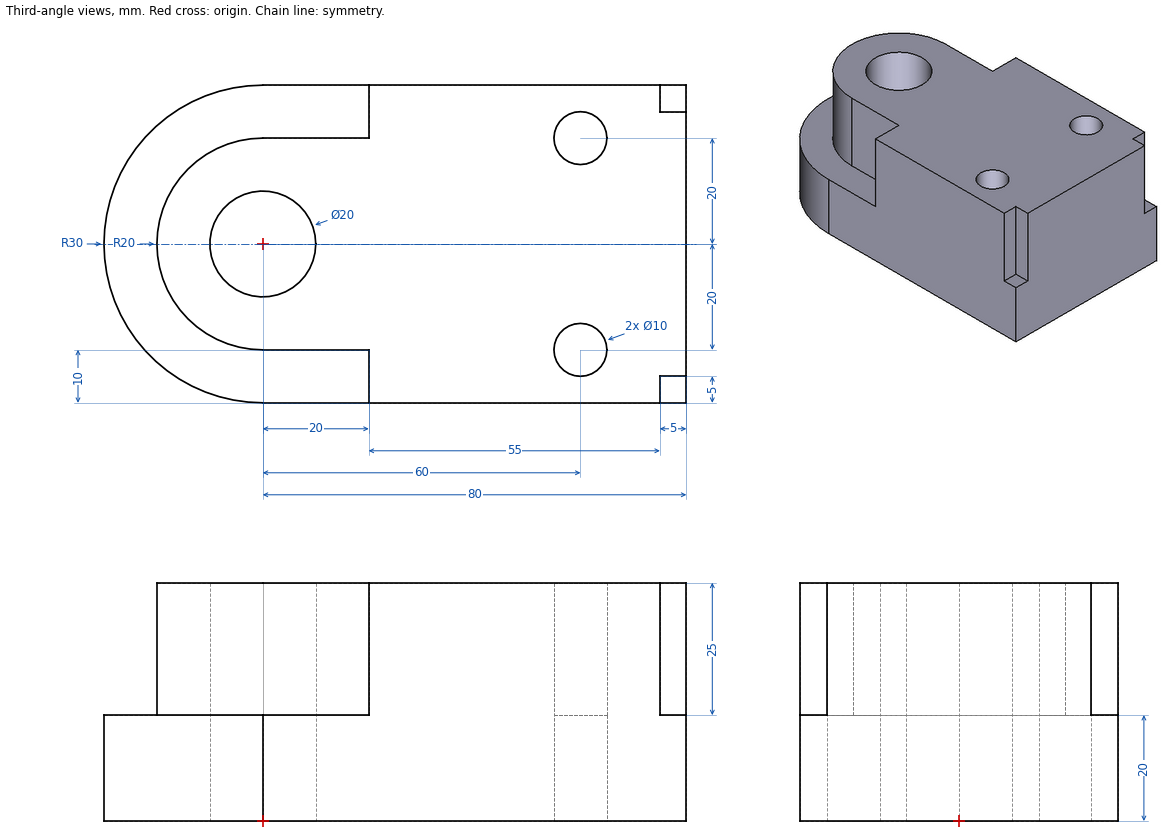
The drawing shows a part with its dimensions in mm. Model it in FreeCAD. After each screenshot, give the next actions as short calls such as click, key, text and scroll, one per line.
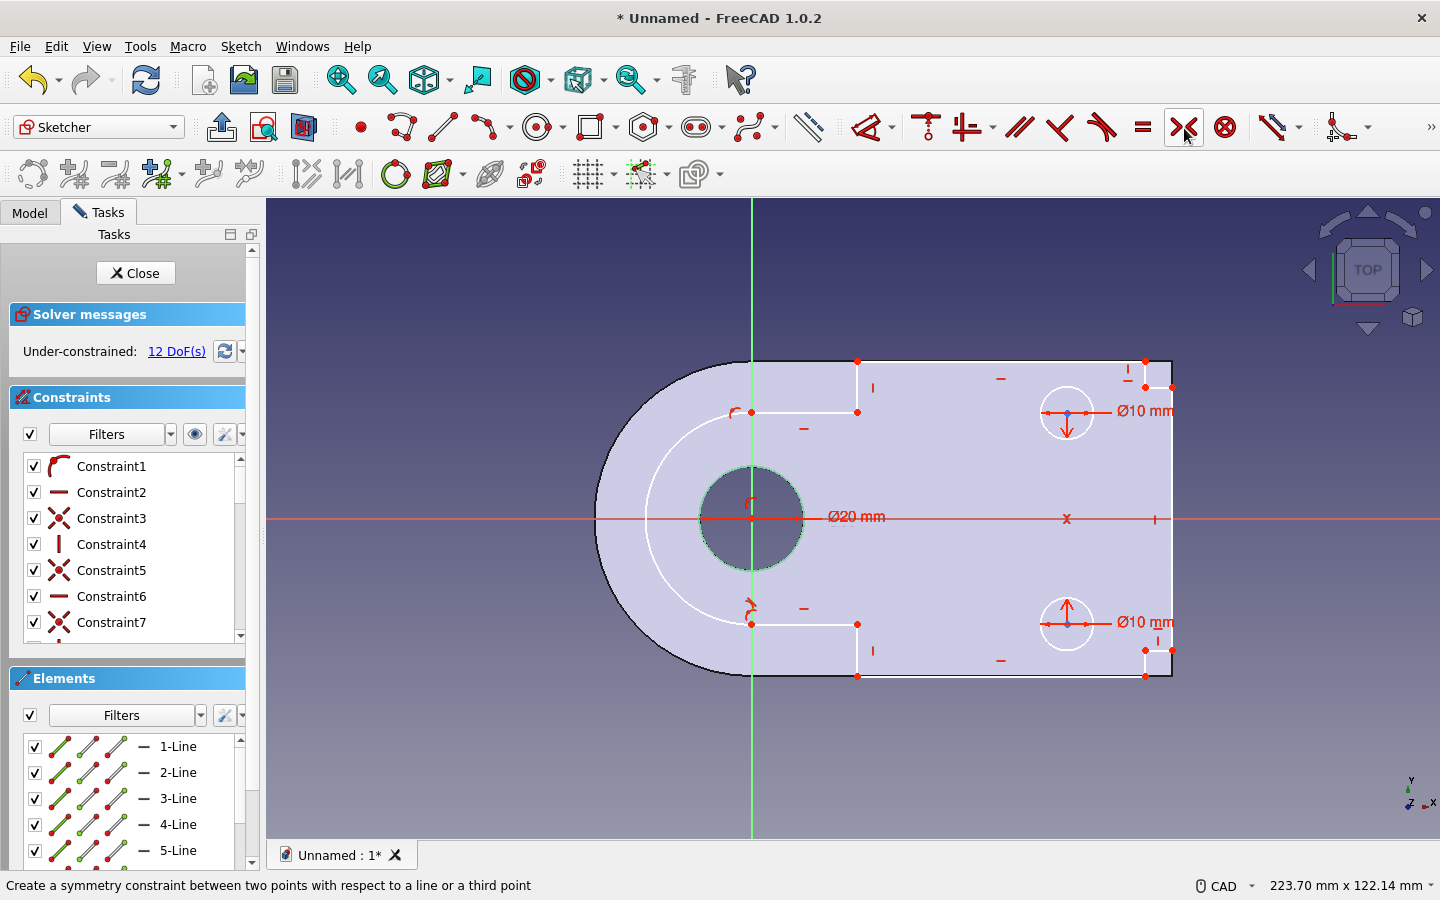
click(1145, 651)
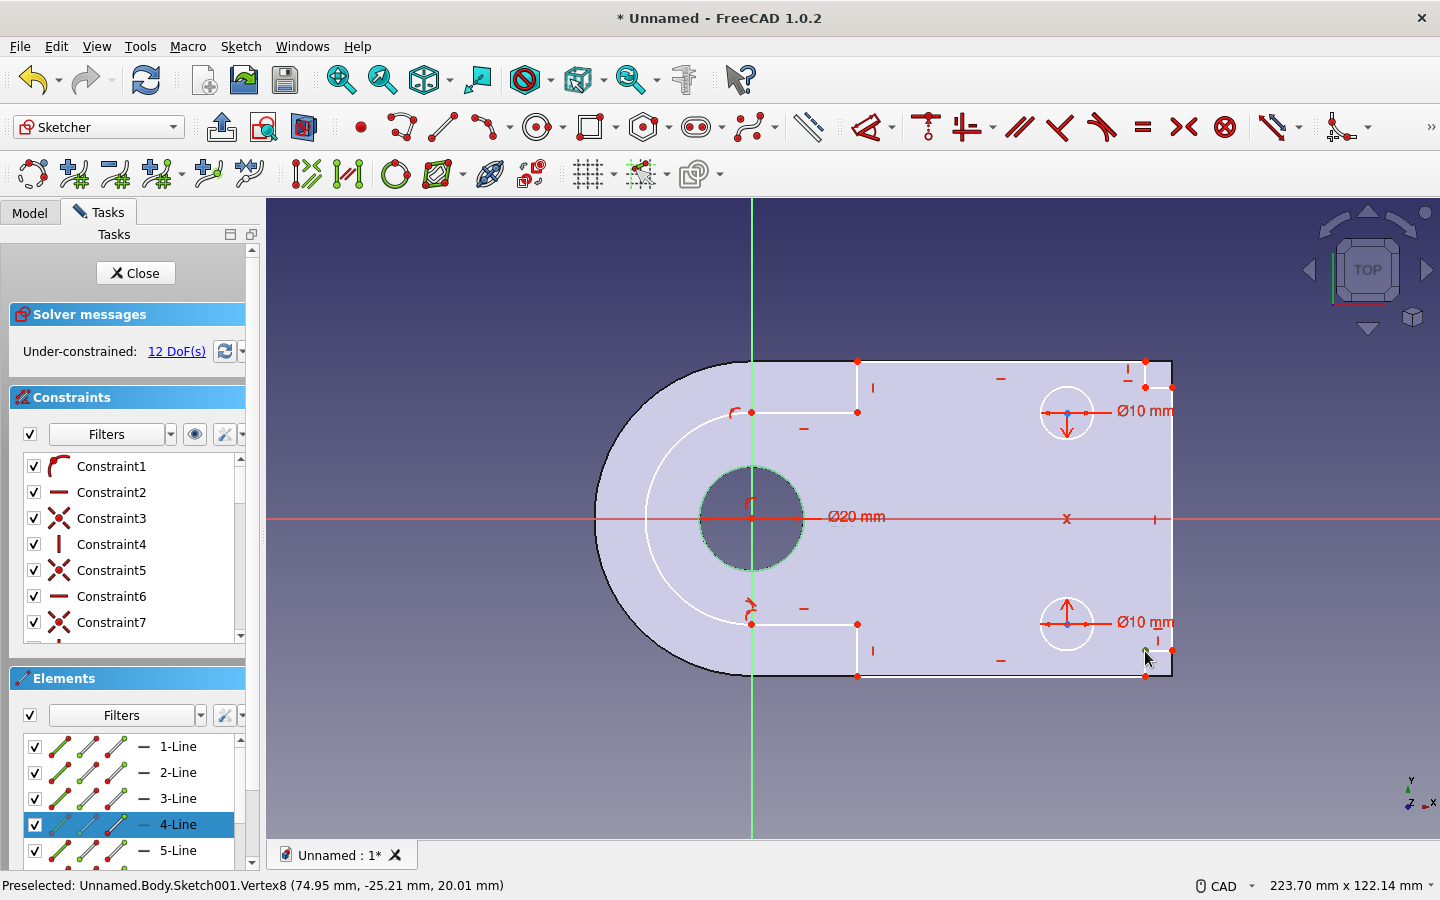
click(1145, 388)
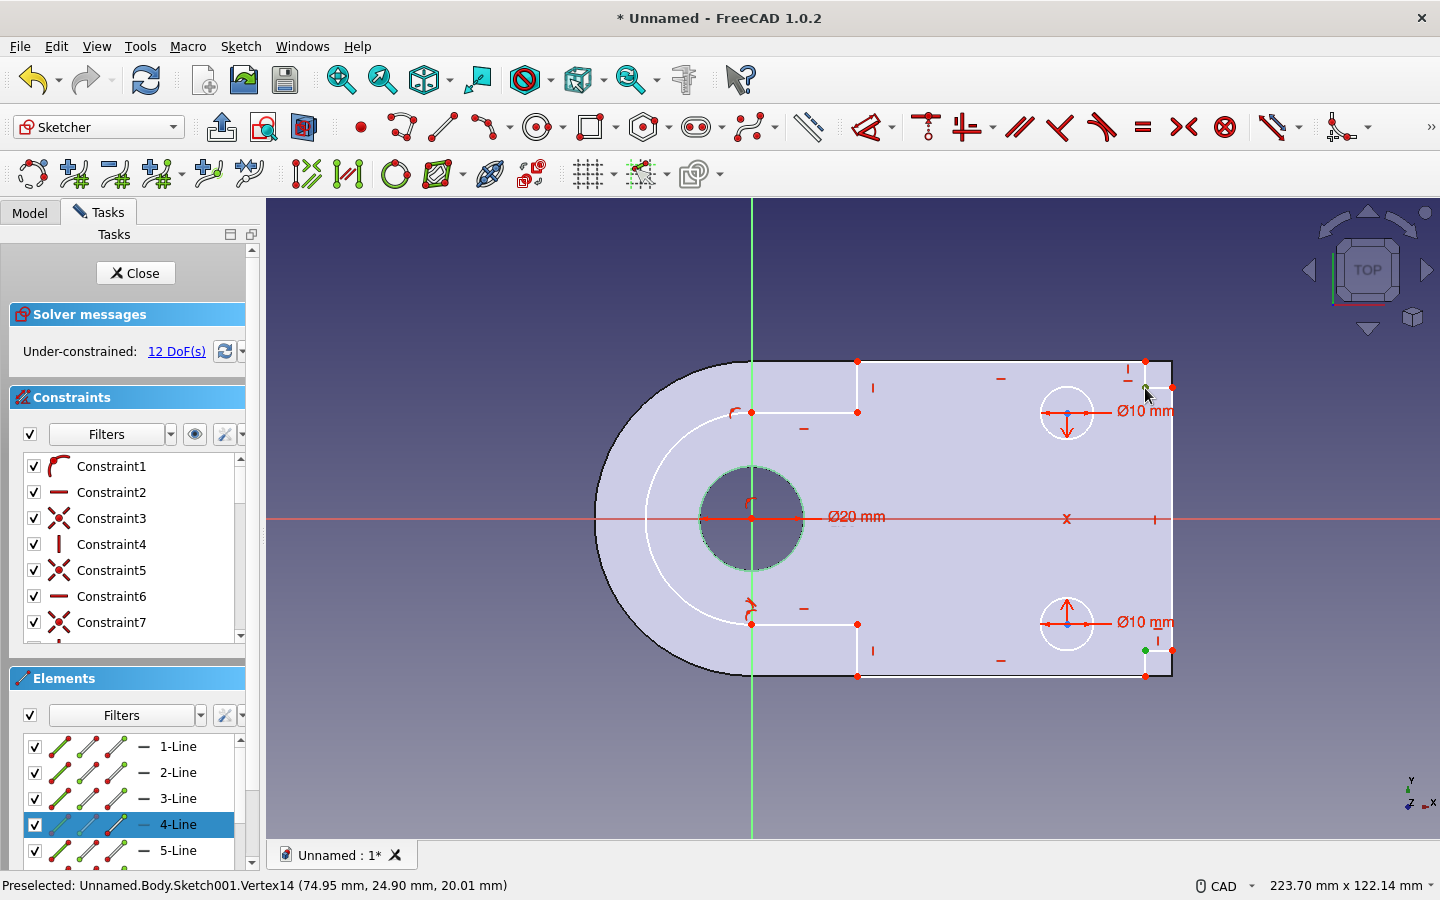
click(364, 519)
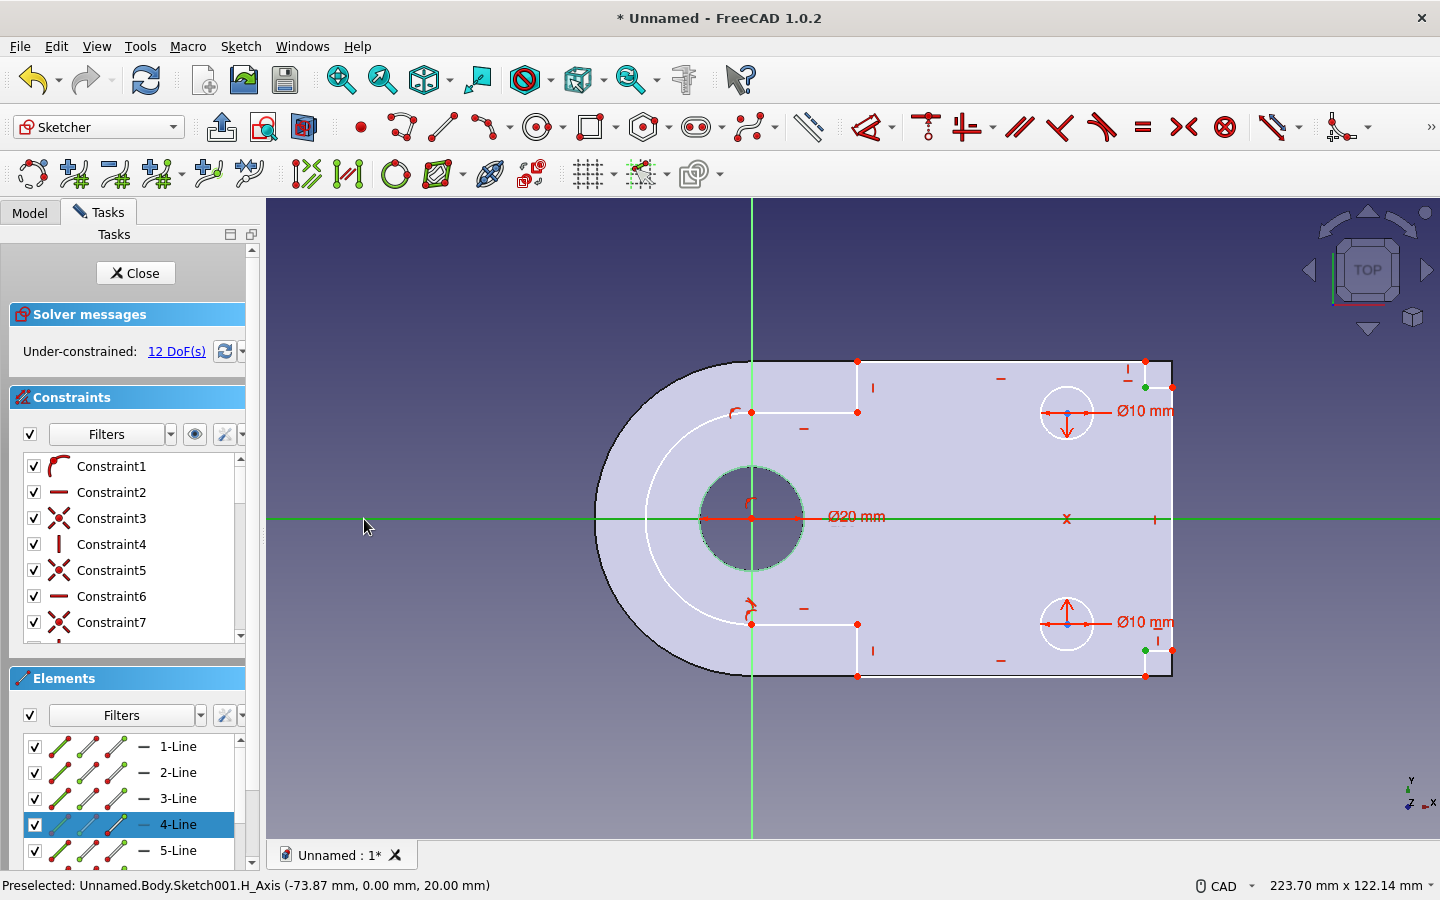
key(s)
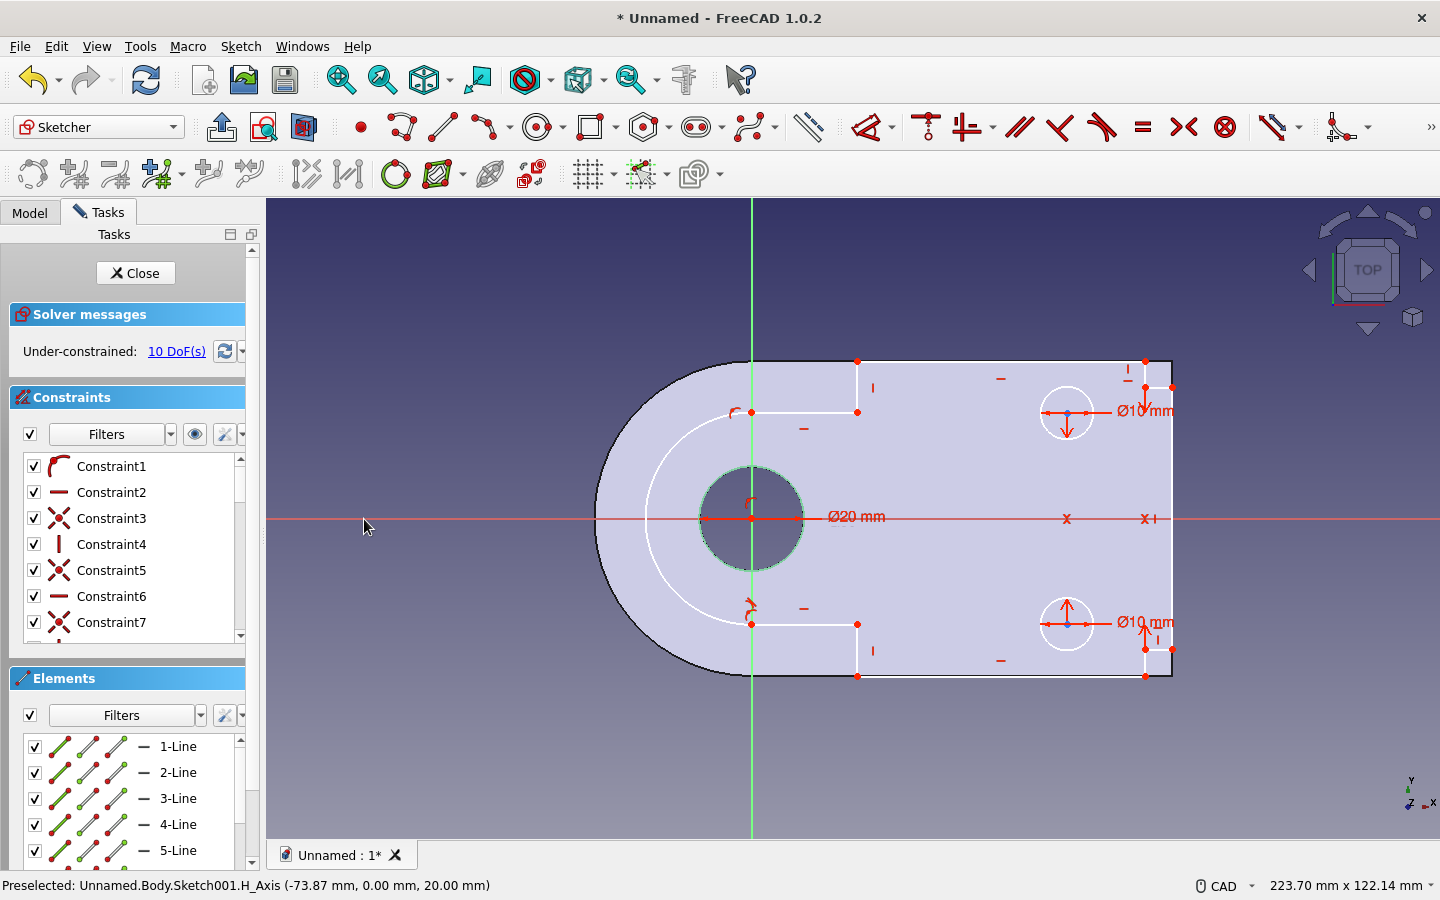
click(857, 677)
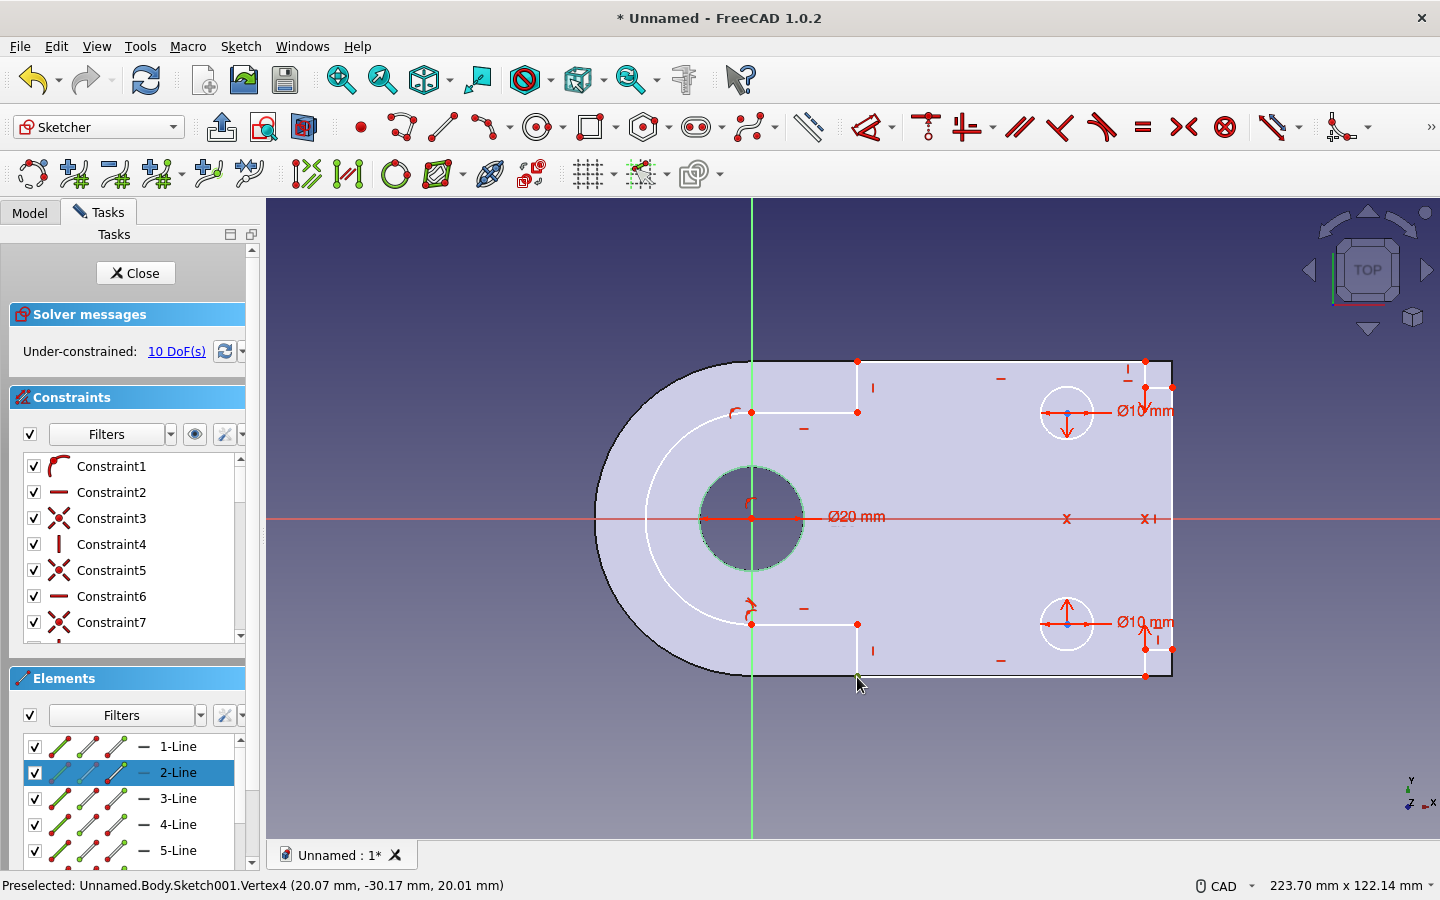
click(857, 362)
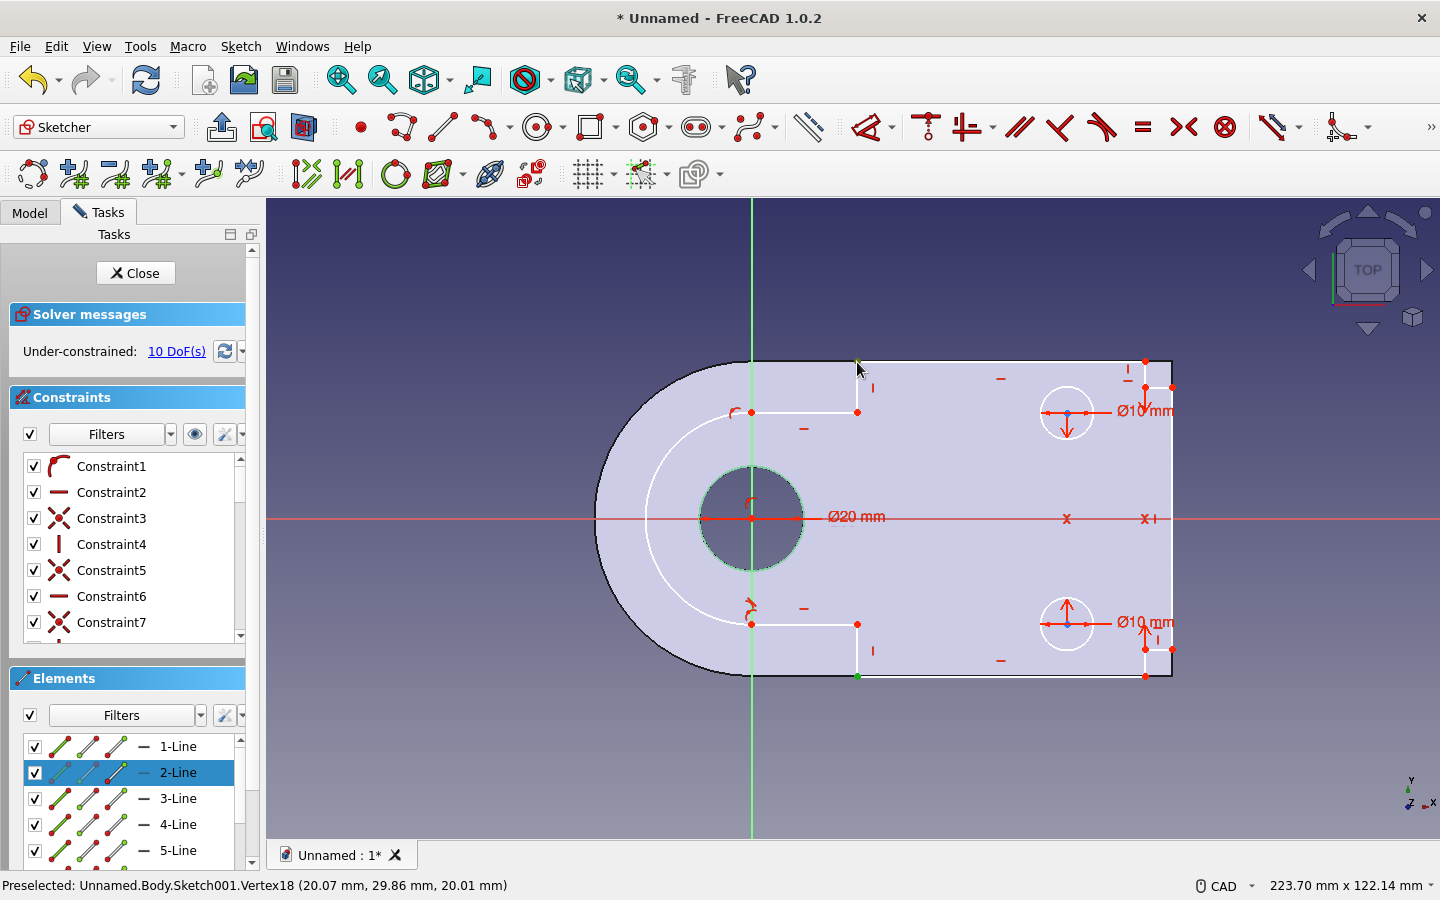
click(364, 519)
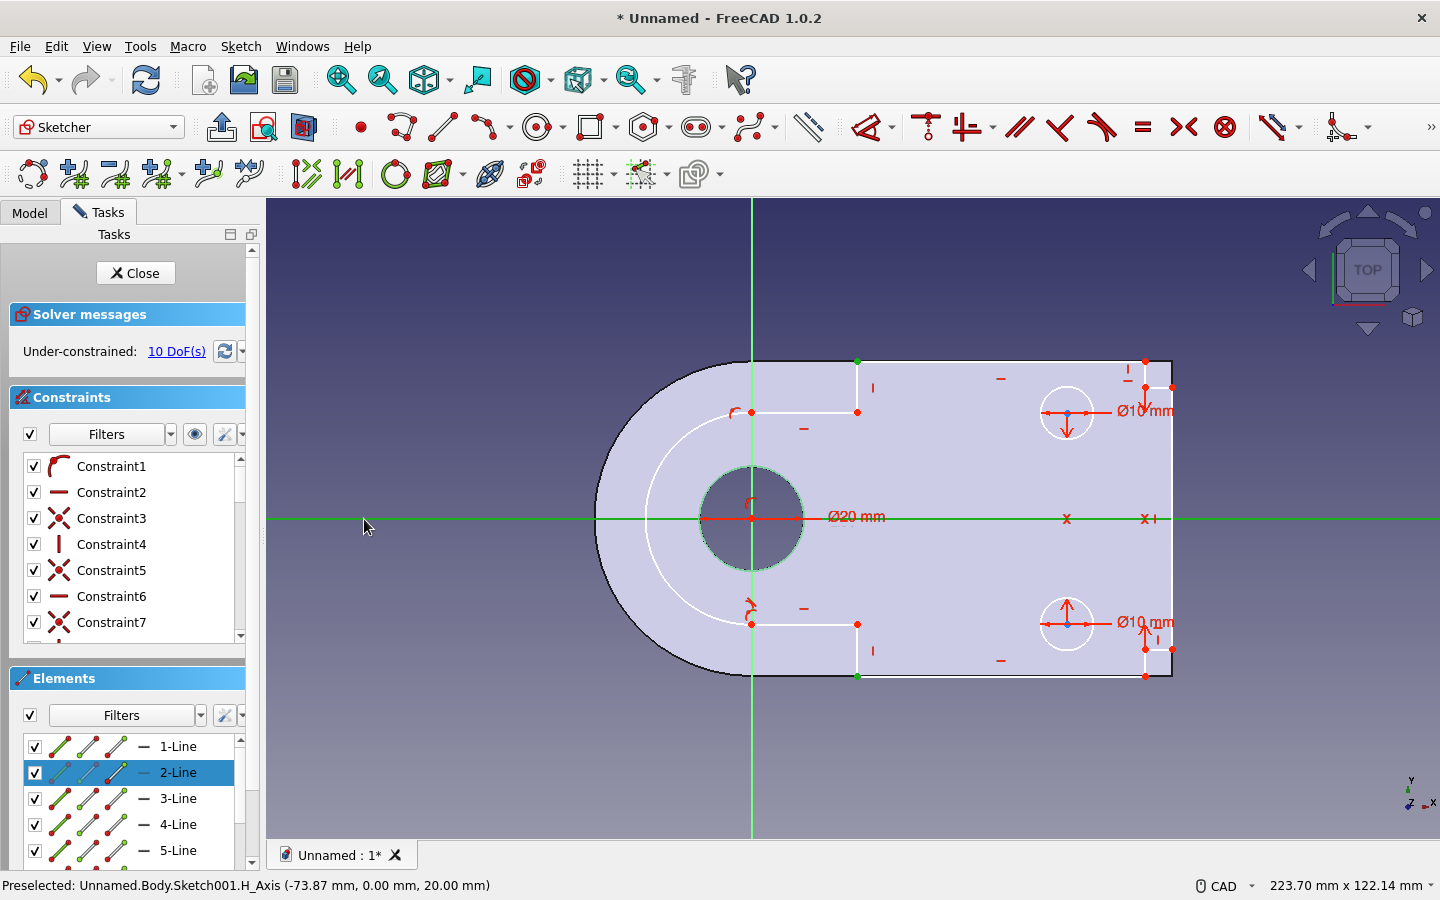
click(1184, 128)